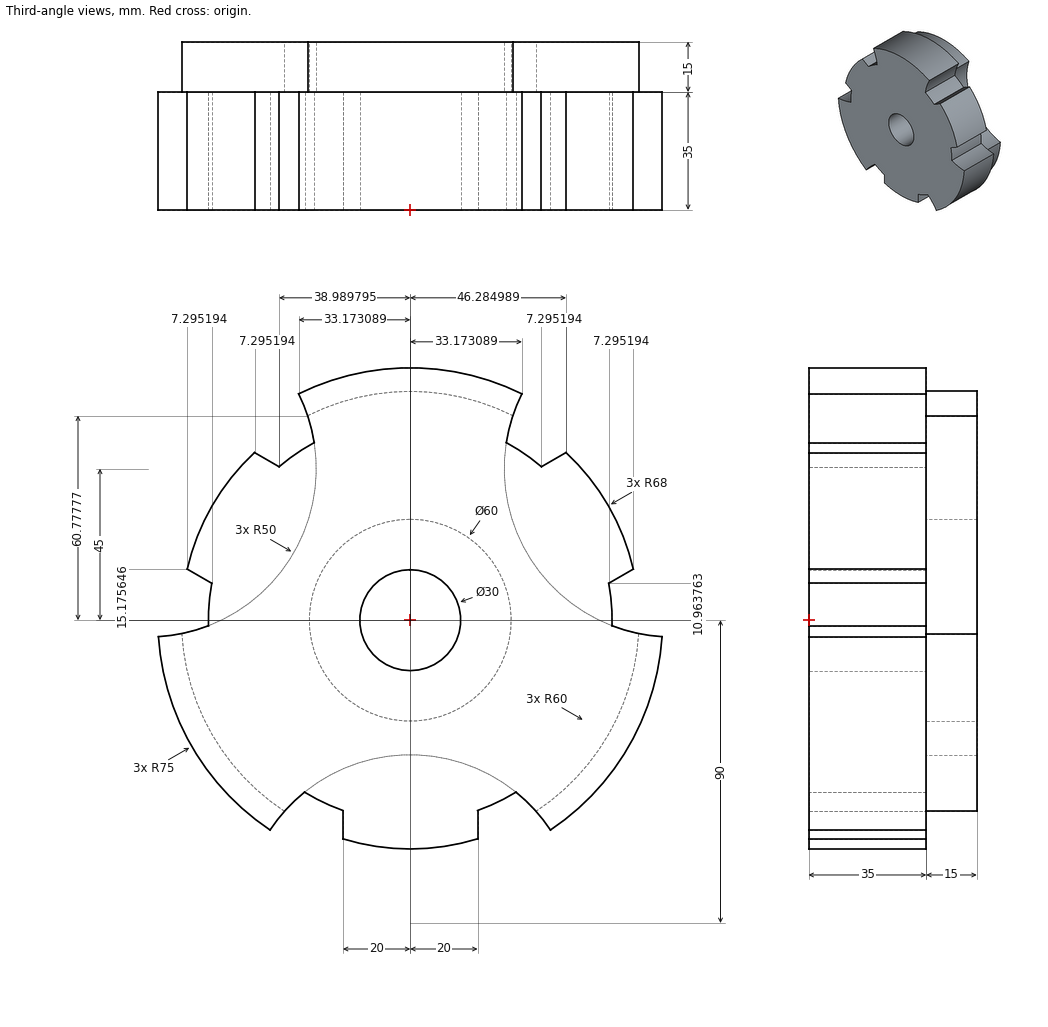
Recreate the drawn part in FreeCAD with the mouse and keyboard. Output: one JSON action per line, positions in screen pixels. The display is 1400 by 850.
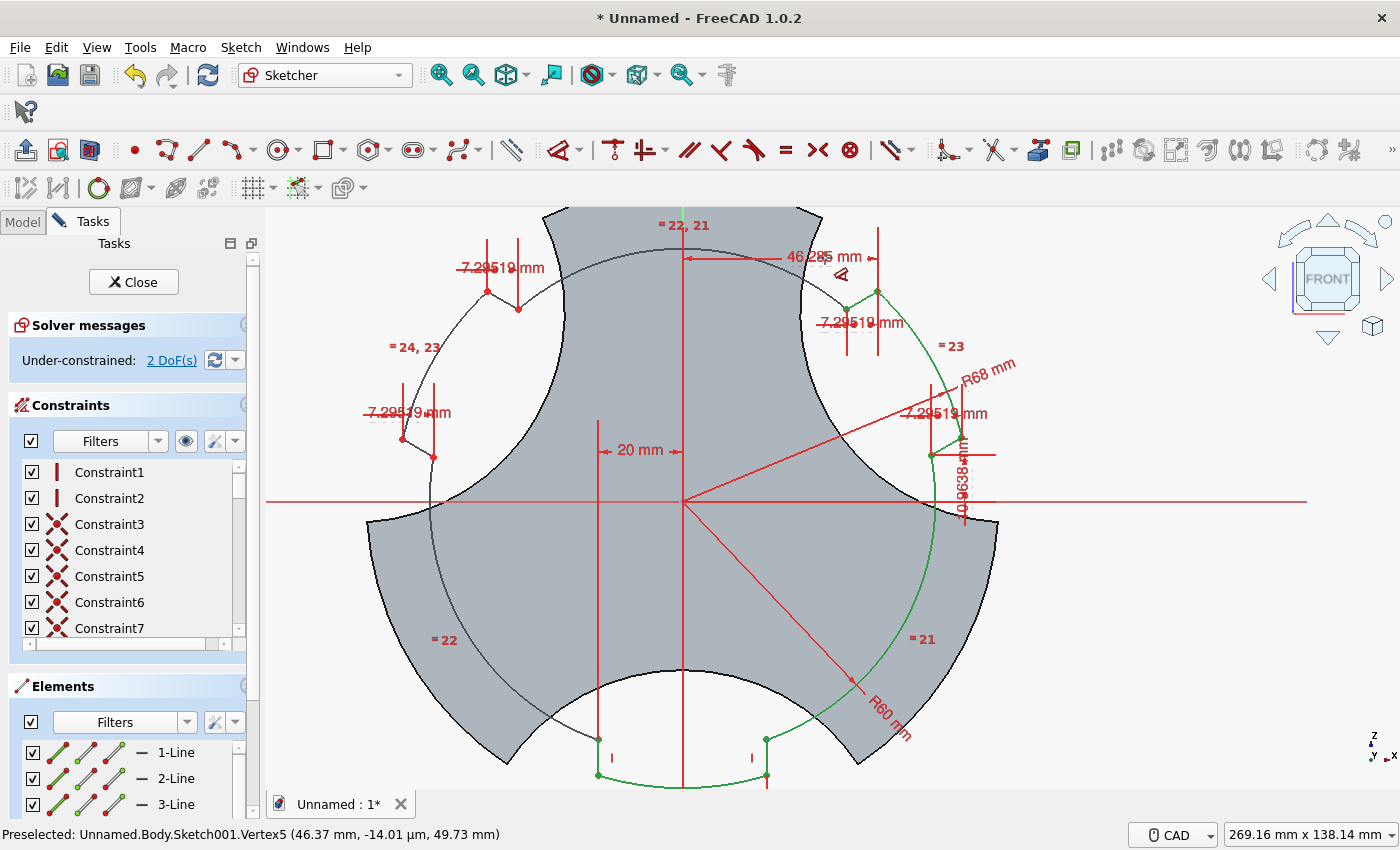
{"action": "left_click", "coordinate": [518, 309]}
{"action": "left_click", "coordinate": [638, 275]}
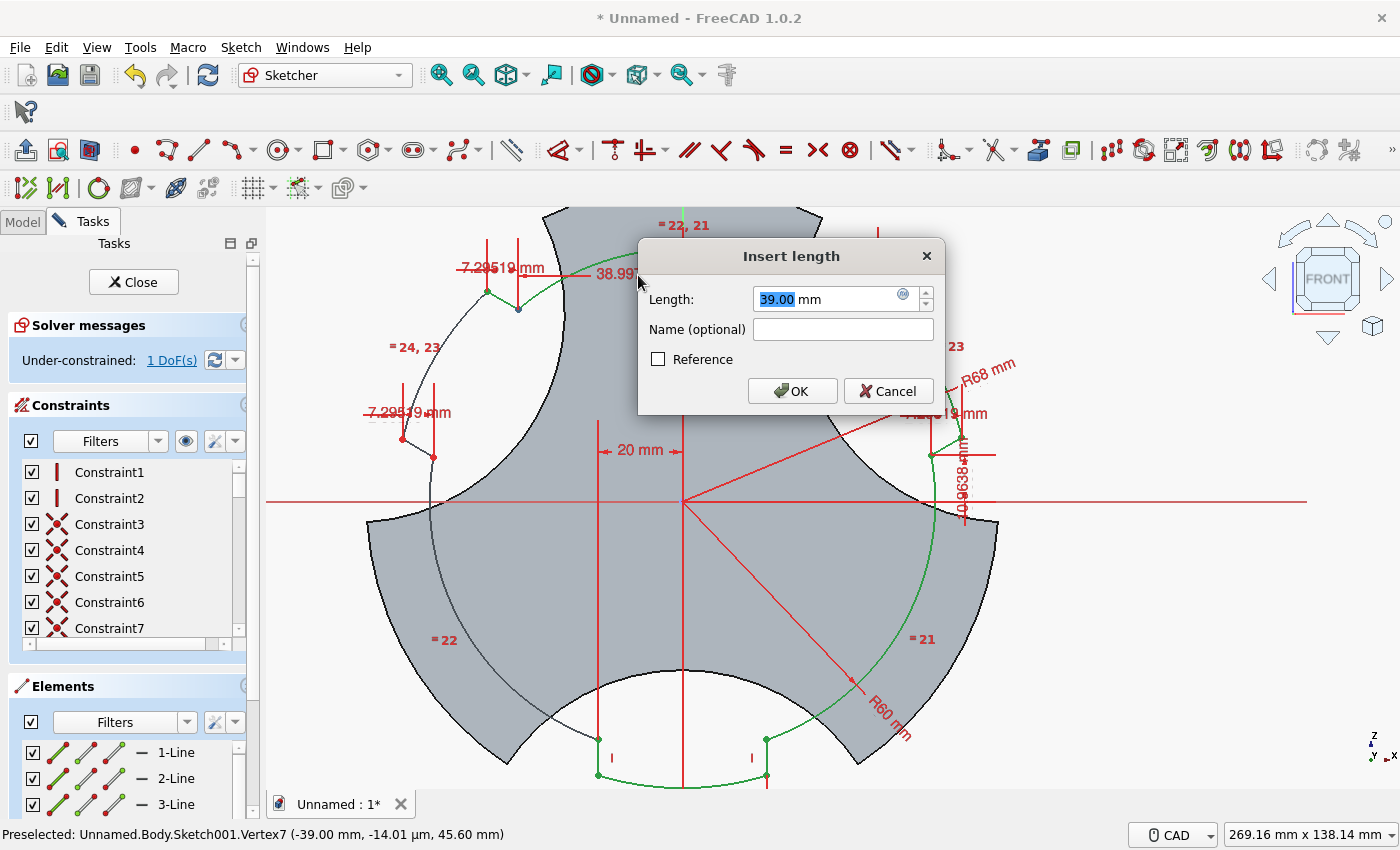
{"action": "type", "text": "38.989795"}
{"action": "key", "text": "Return"}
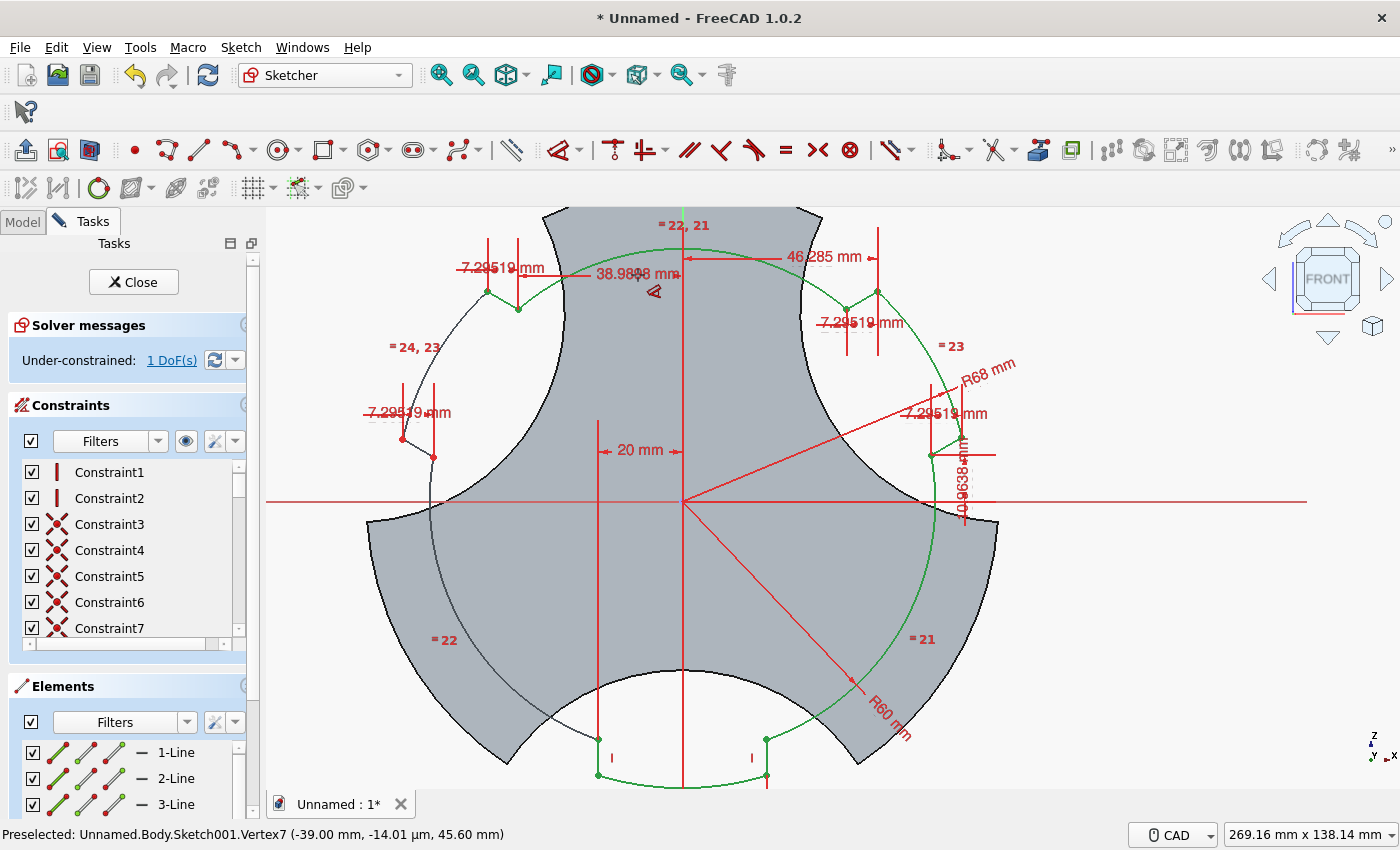
{"action": "left_click", "coordinate": [403, 439]}
{"action": "left_click", "coordinate": [369, 470]}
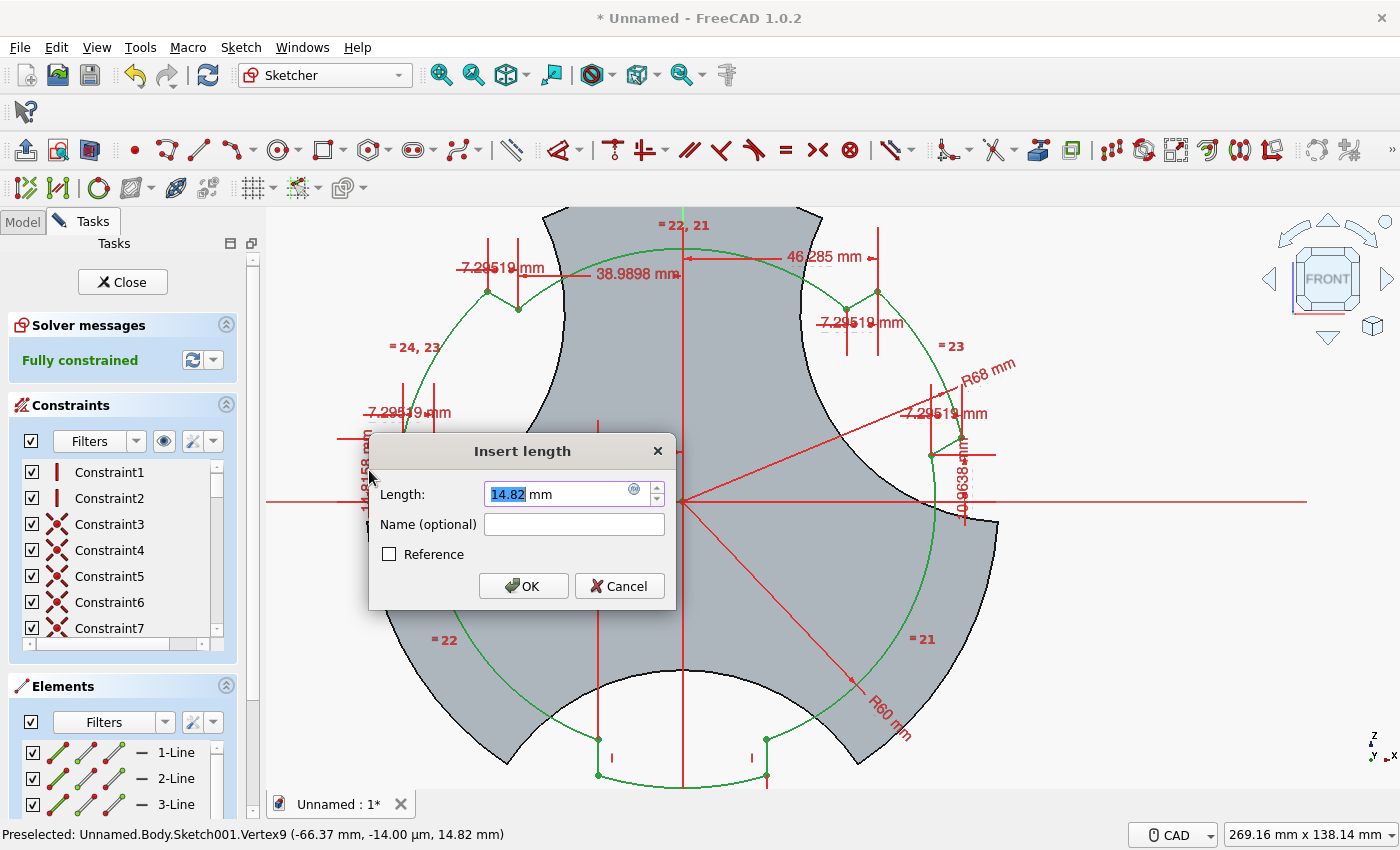
{"action": "type", "text": "15.175646"}
{"action": "key", "text": "Return"}
{"action": "key", "text": "Escape"}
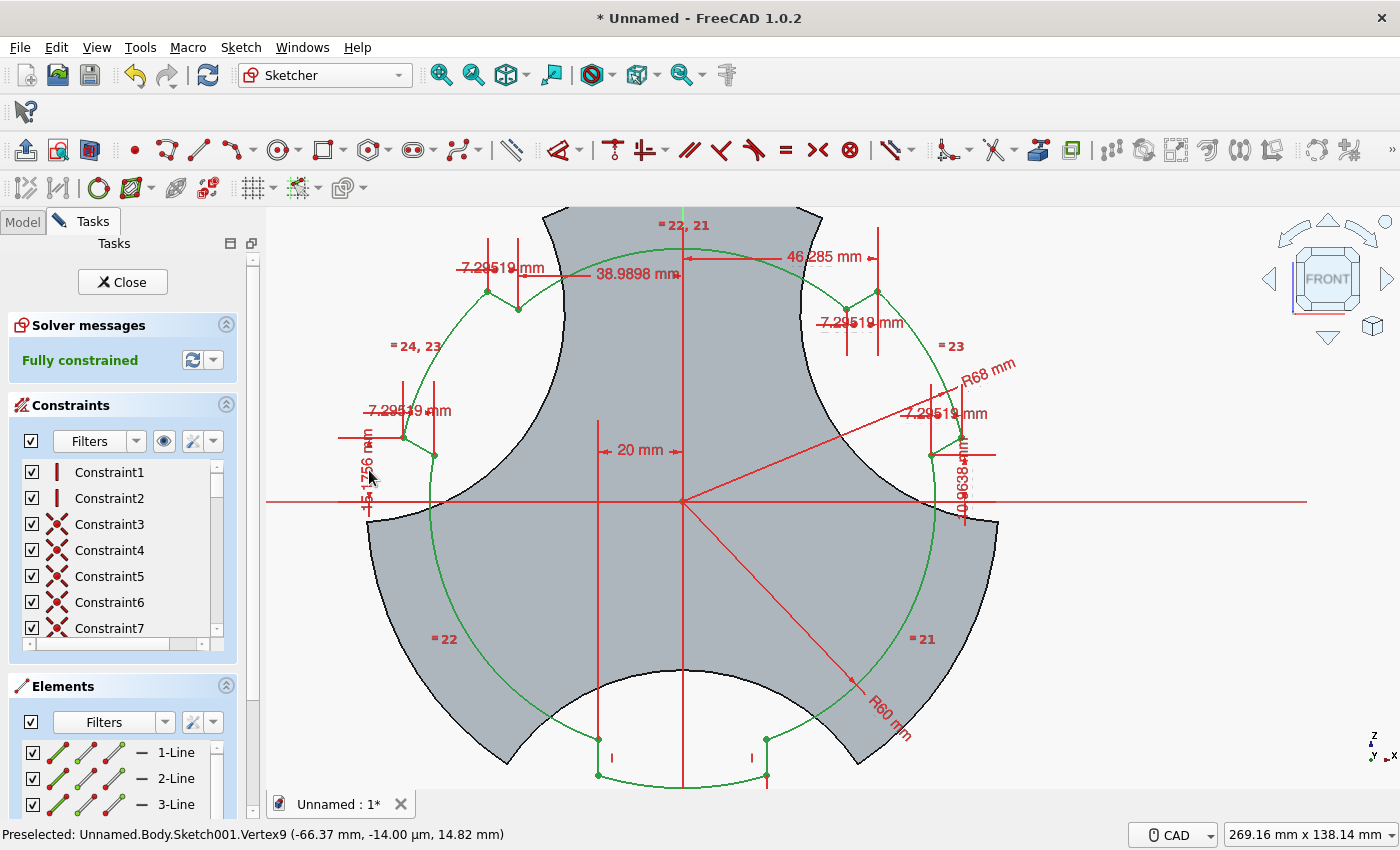
{"action": "left_click", "coordinate": [123, 282]}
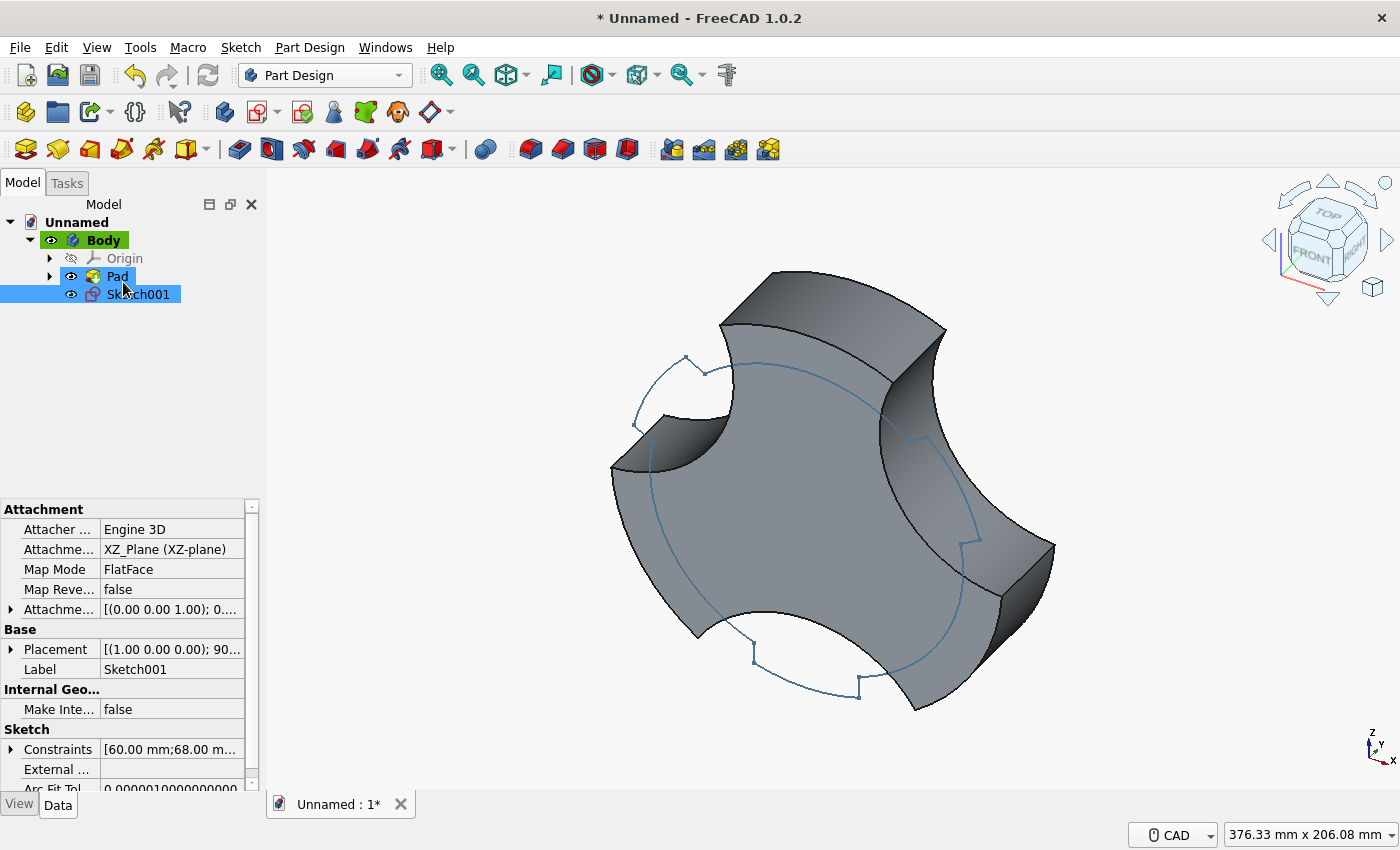
{"action": "left_click", "coordinate": [26, 150]}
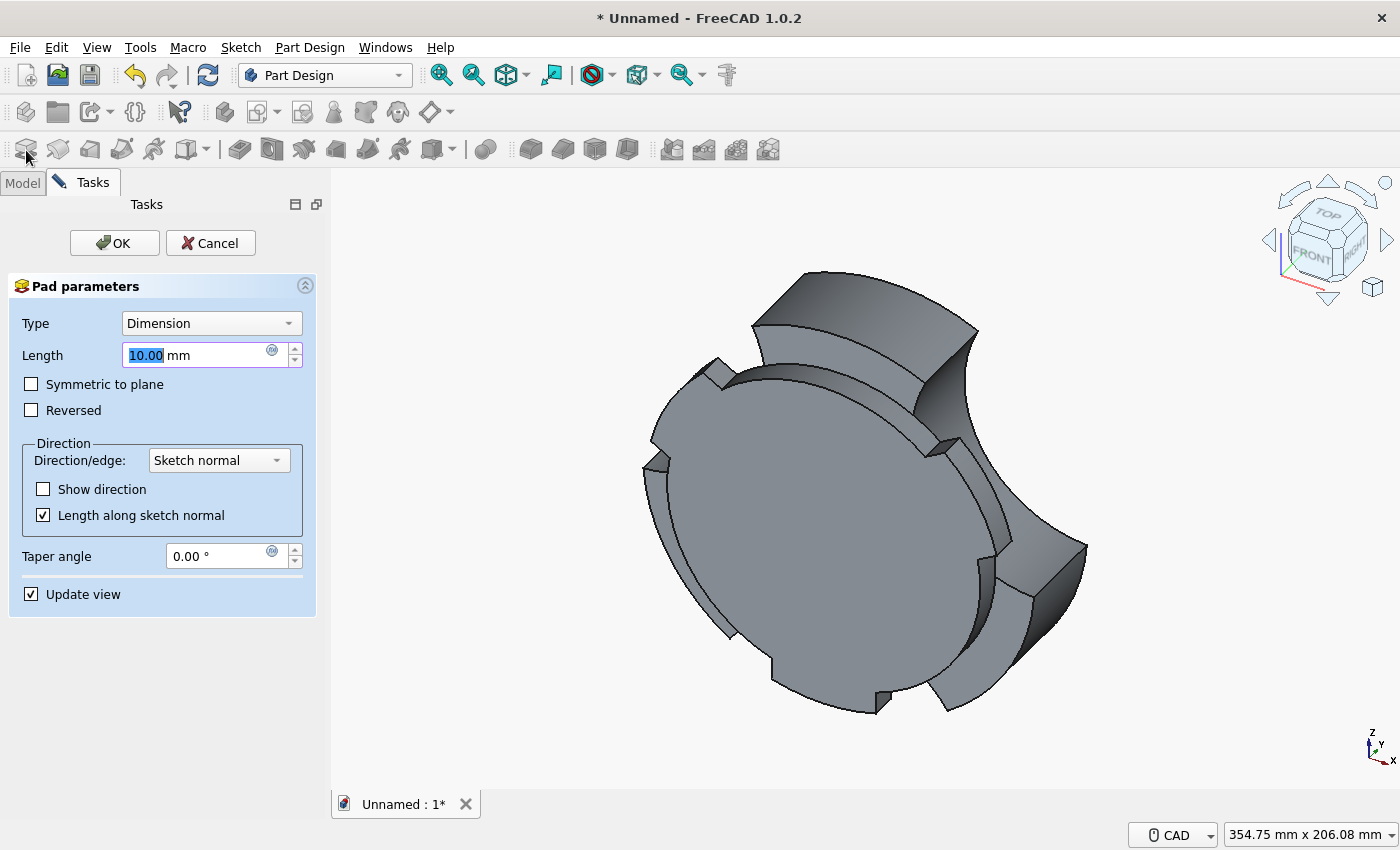
{"action": "type", "text": "35"}
{"action": "key", "text": "Tab"}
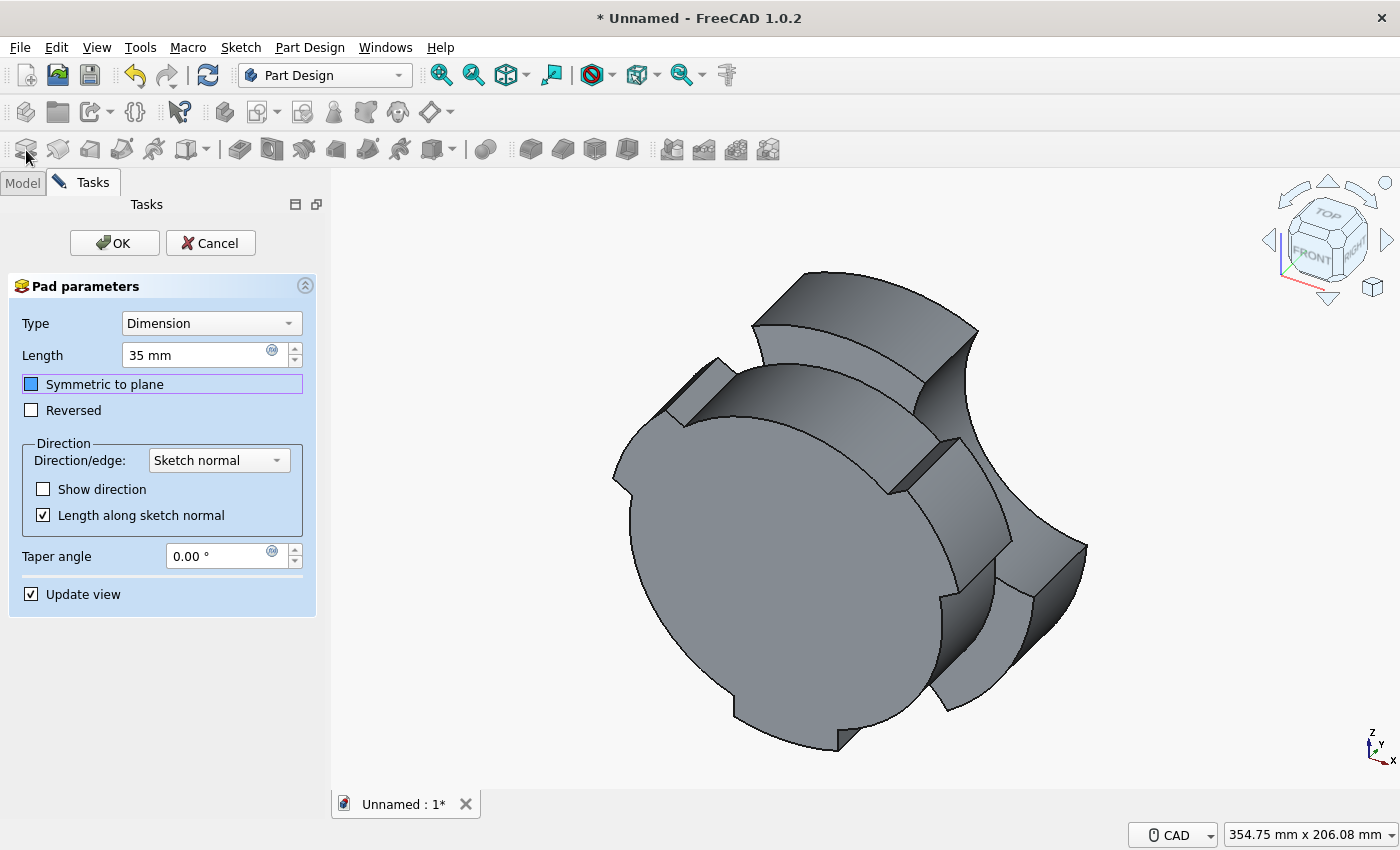
{"action": "left_click", "coordinate": [30, 410]}